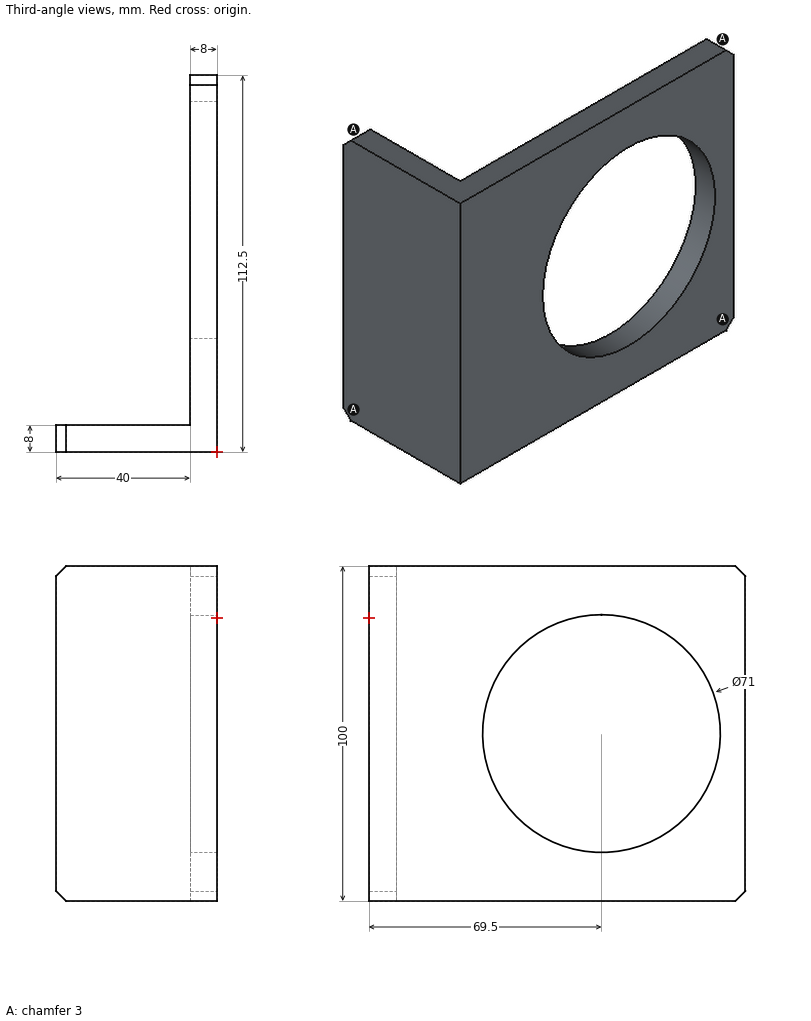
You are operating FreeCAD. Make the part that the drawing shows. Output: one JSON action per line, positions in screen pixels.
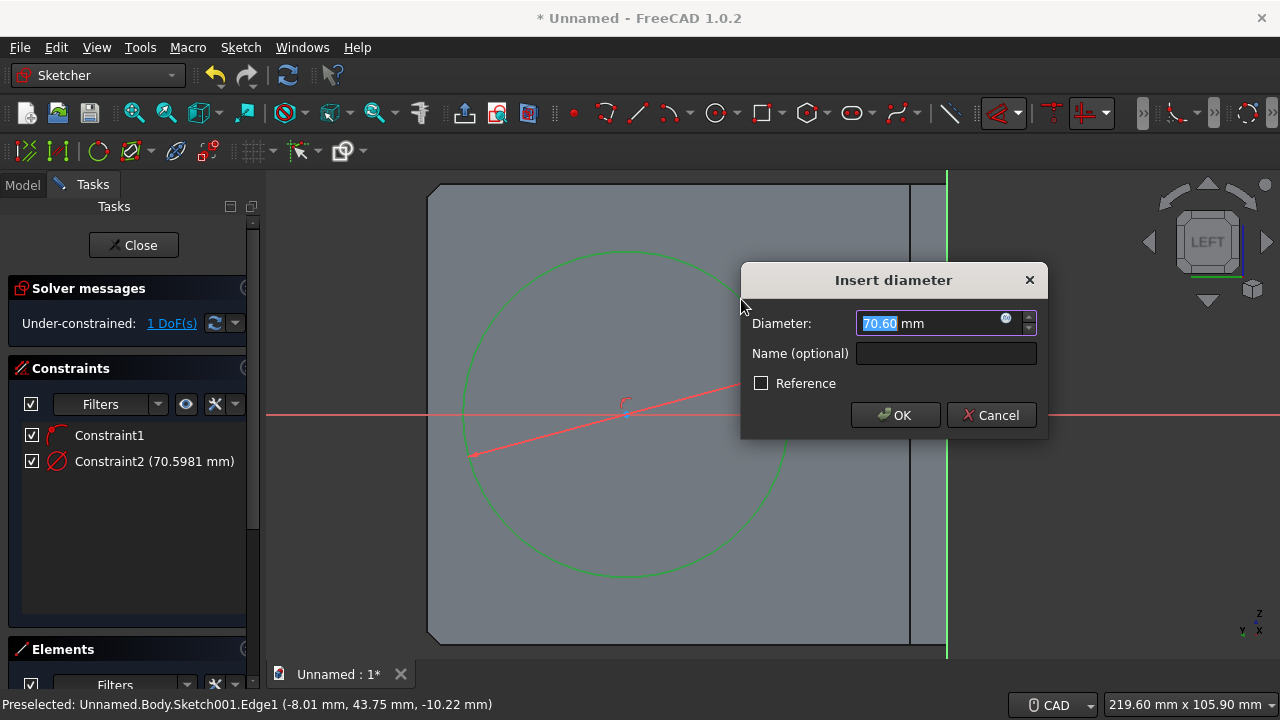
{"action": "type", "text": "71"}
{"action": "key", "text": "Return"}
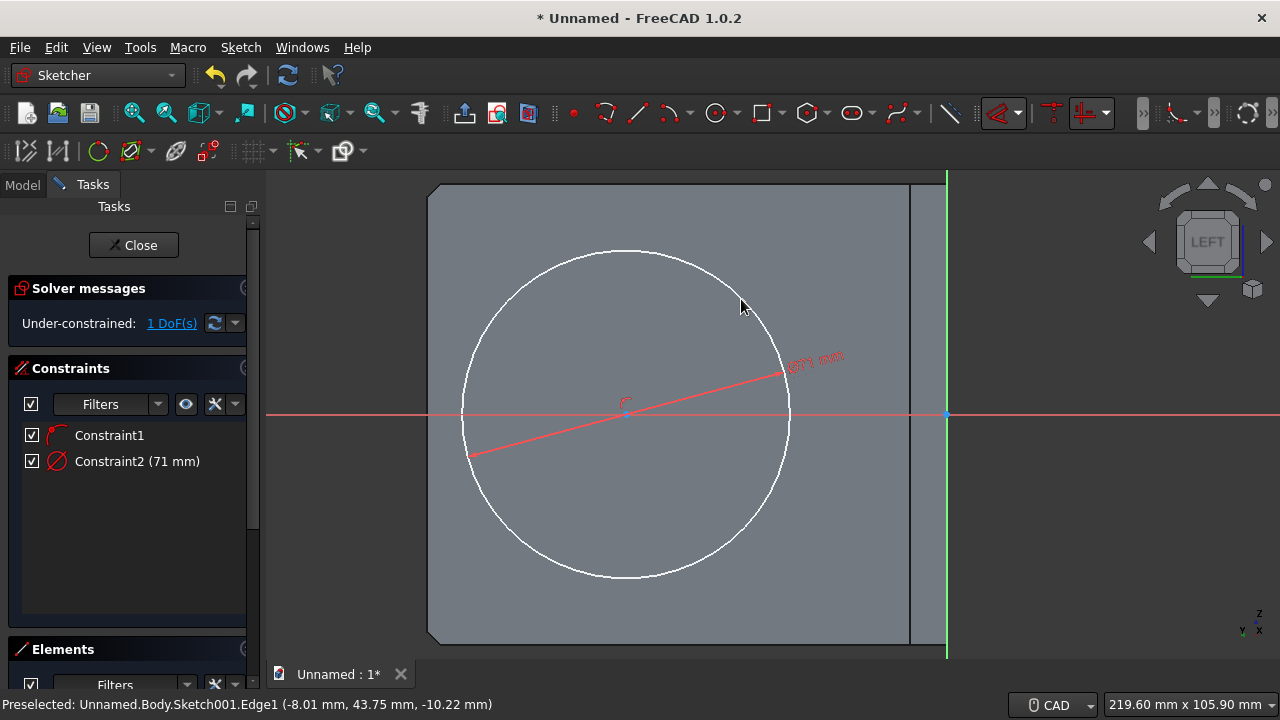
{"action": "left_click", "coordinate": [626, 414]}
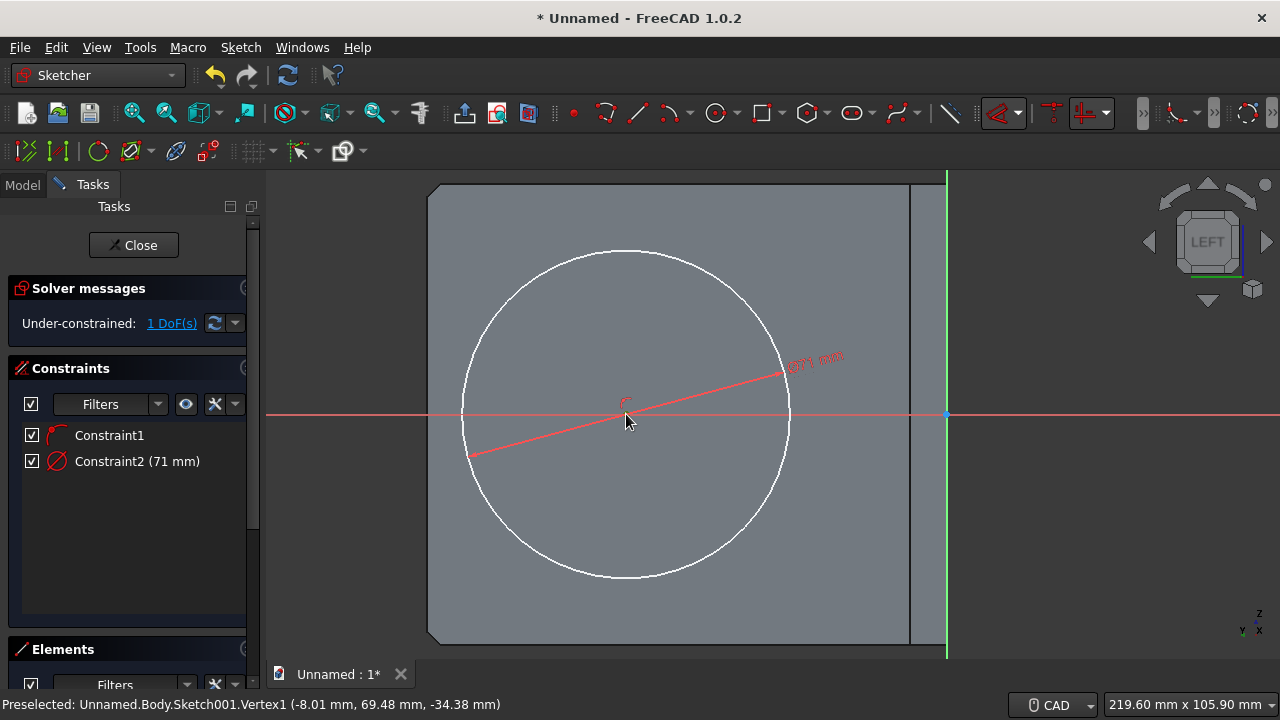
{"action": "left_click", "coordinate": [1020, 114]}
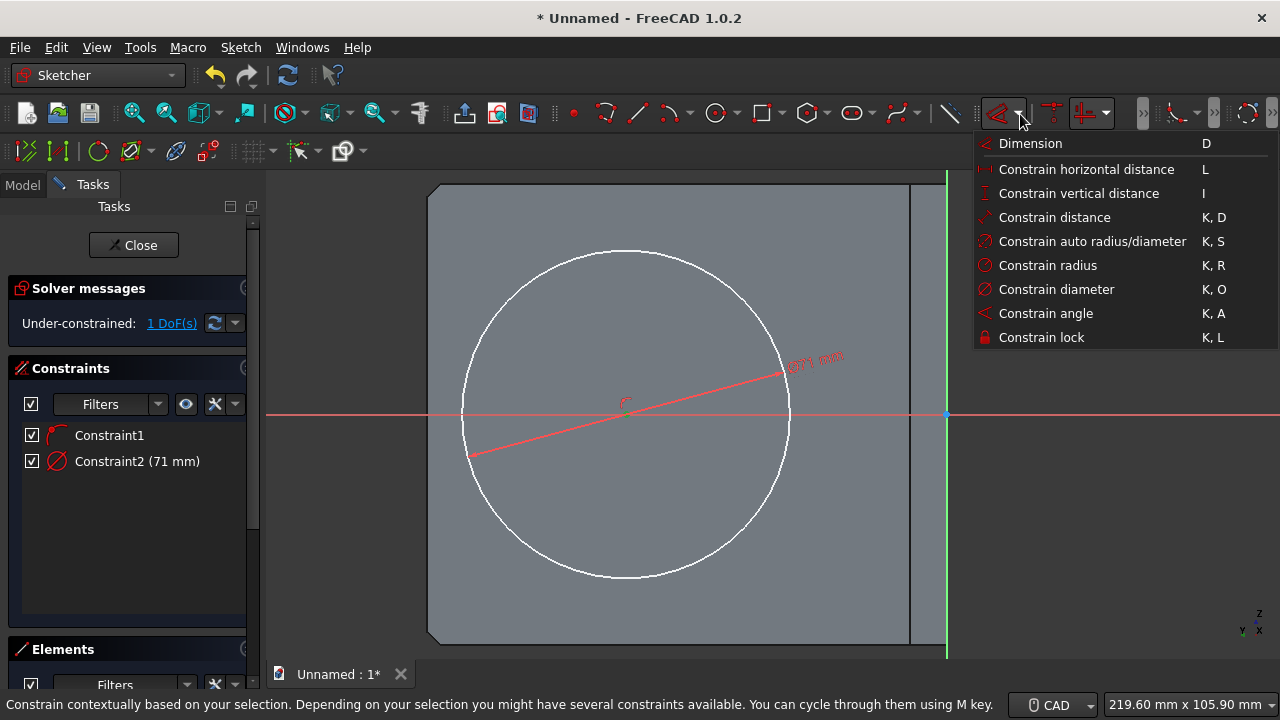
{"action": "left_click", "coordinate": [1126, 169]}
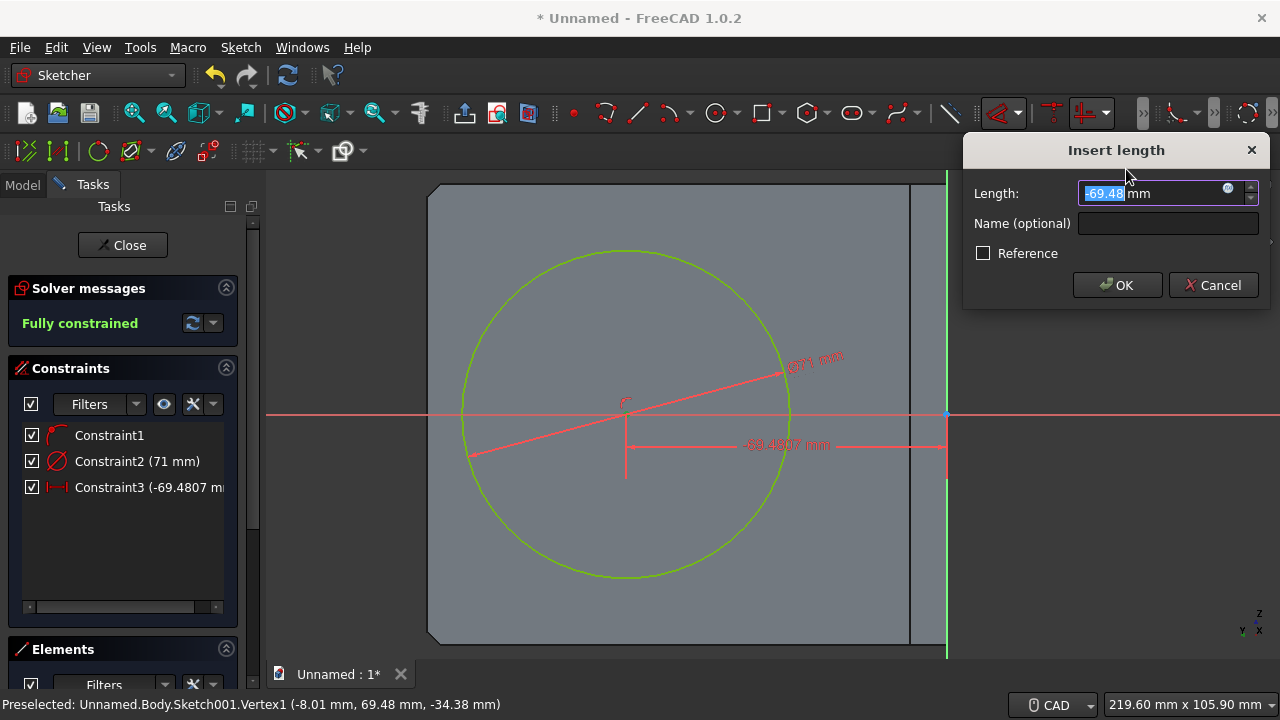
{"action": "type", "text": "-69.5"}
{"action": "key", "text": "Return"}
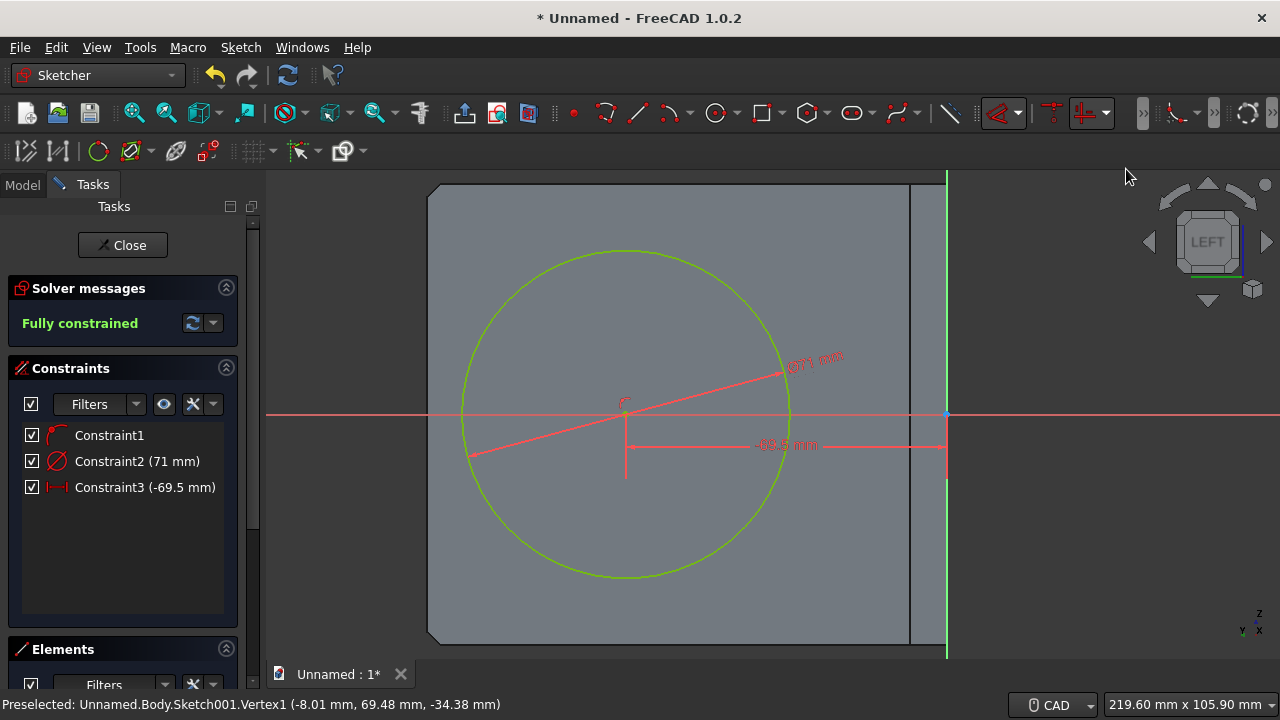
{"action": "left_click", "coordinate": [123, 245]}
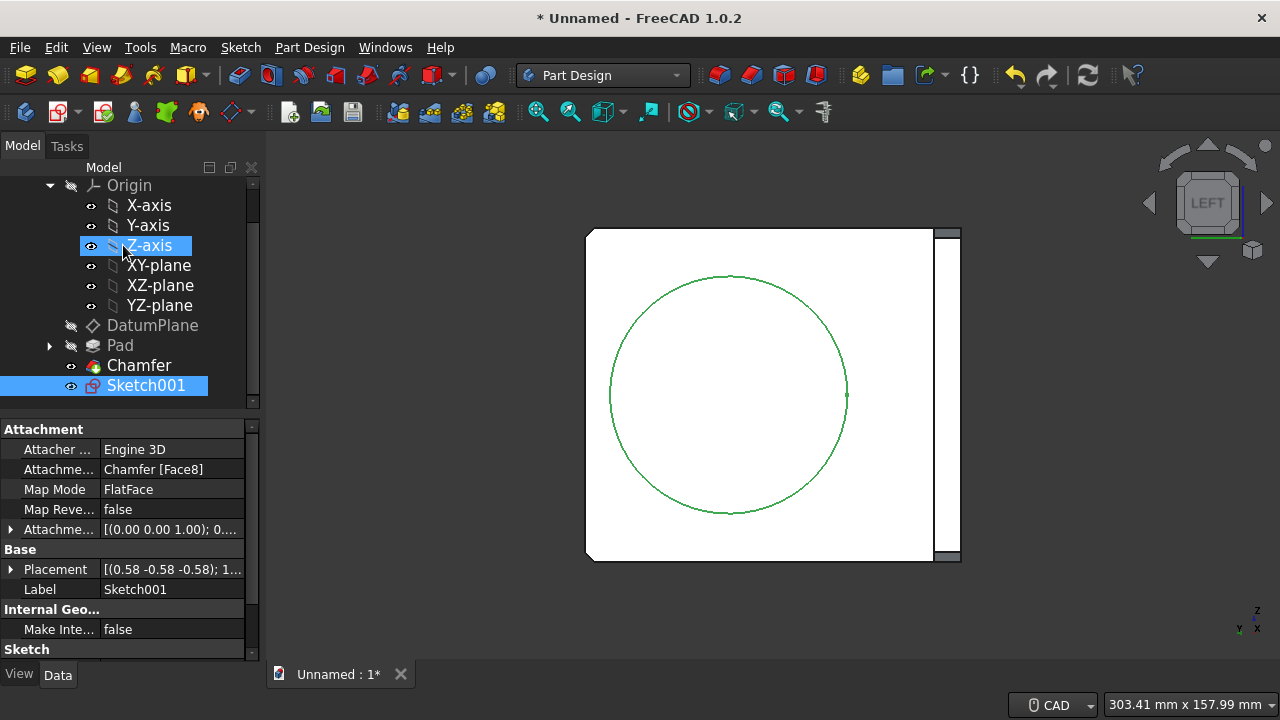
{"action": "left_click", "coordinate": [240, 76]}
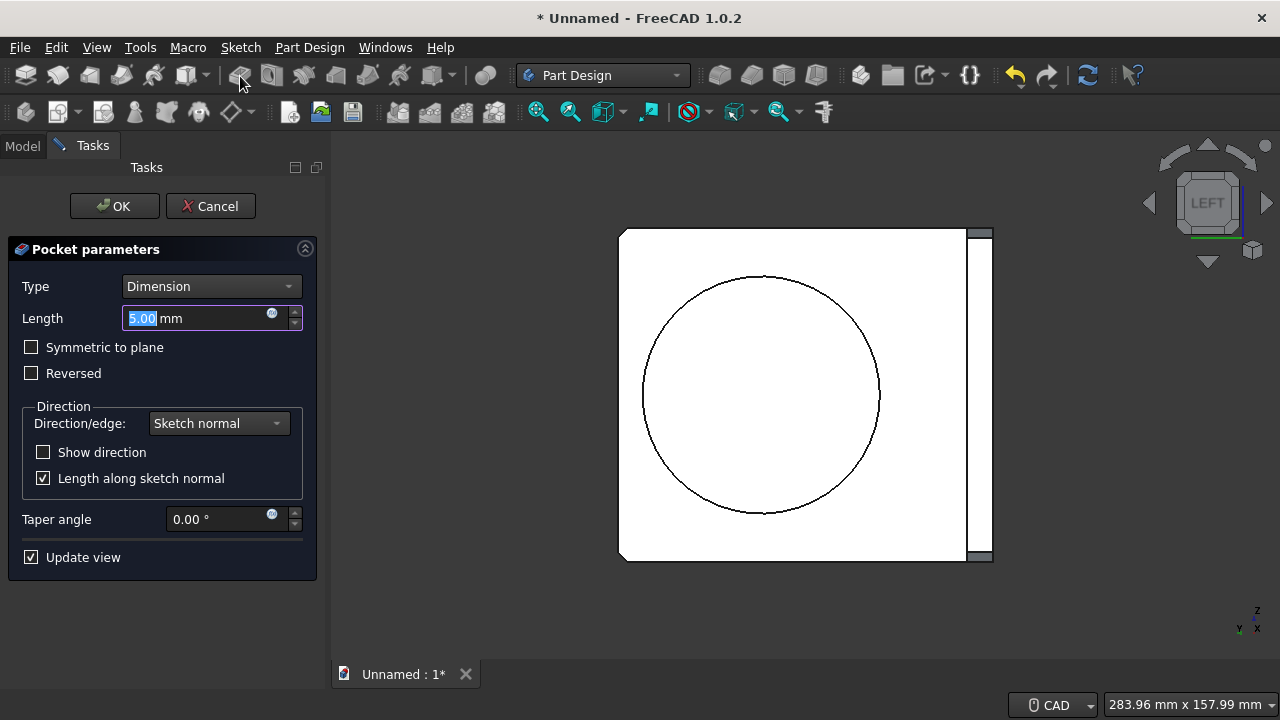
{"action": "left_click", "coordinate": [212, 286]}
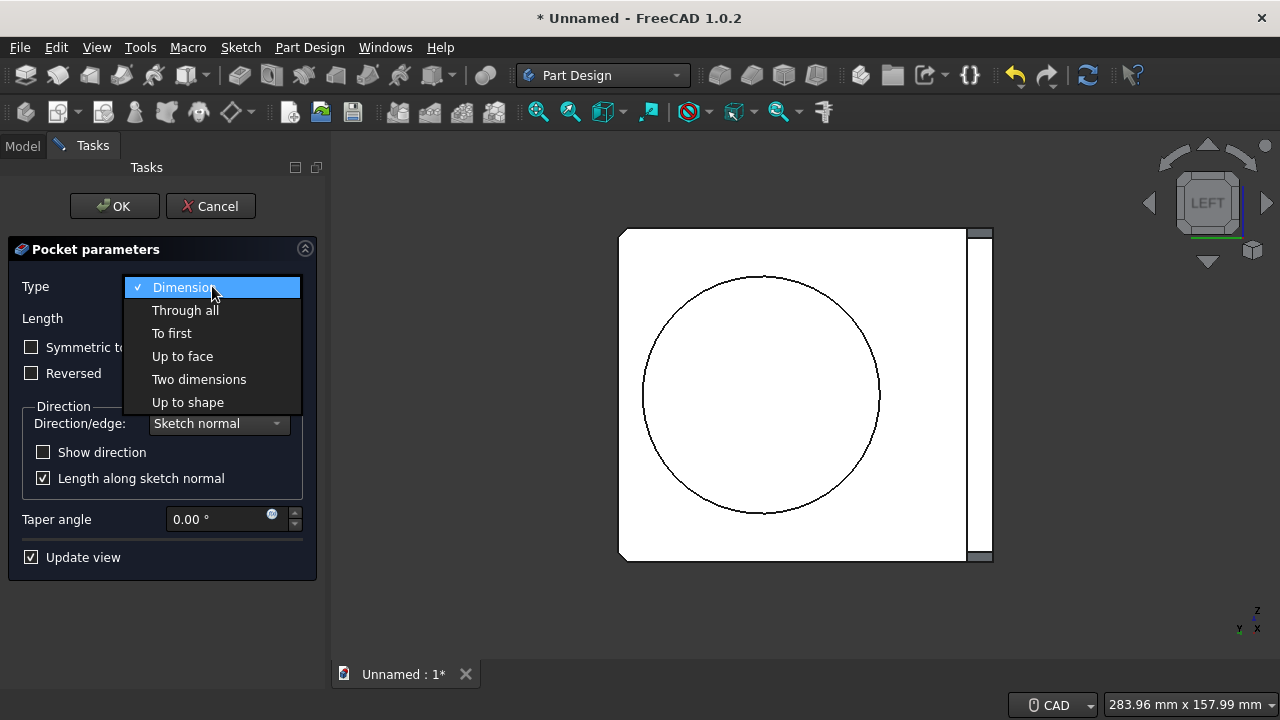
{"action": "left_click", "coordinate": [212, 334]}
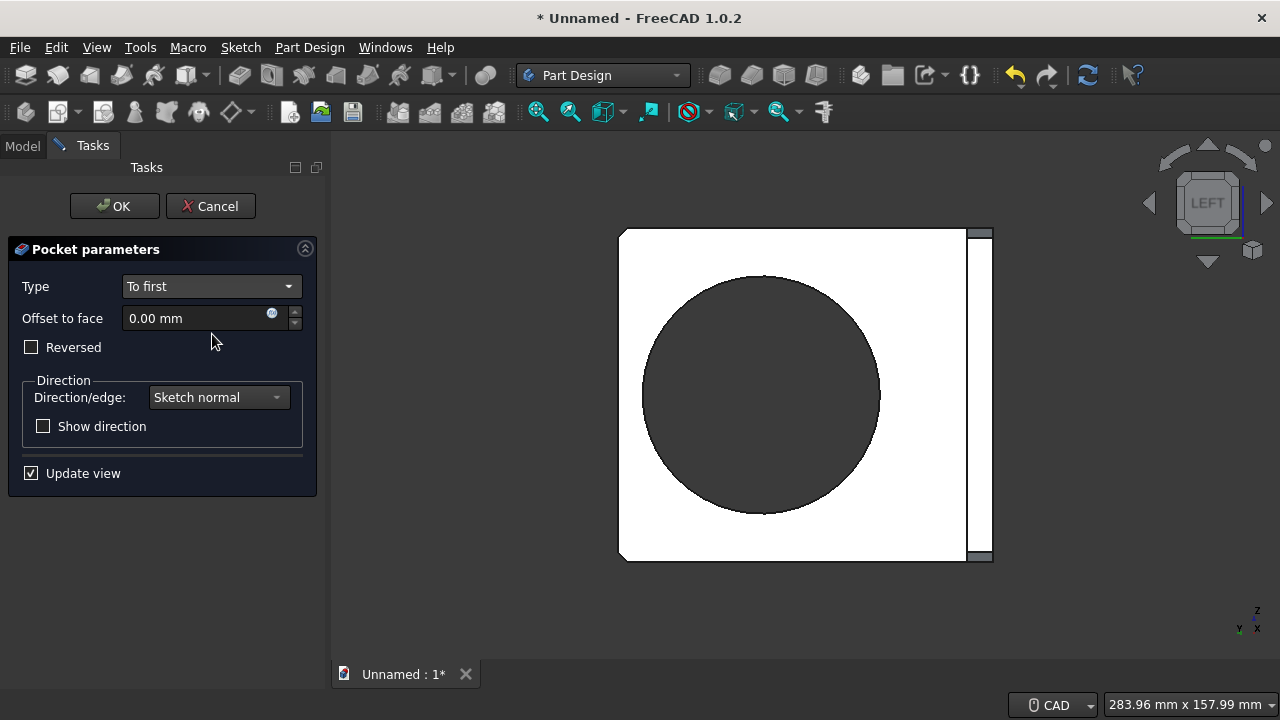
{"action": "left_click", "coordinate": [115, 206]}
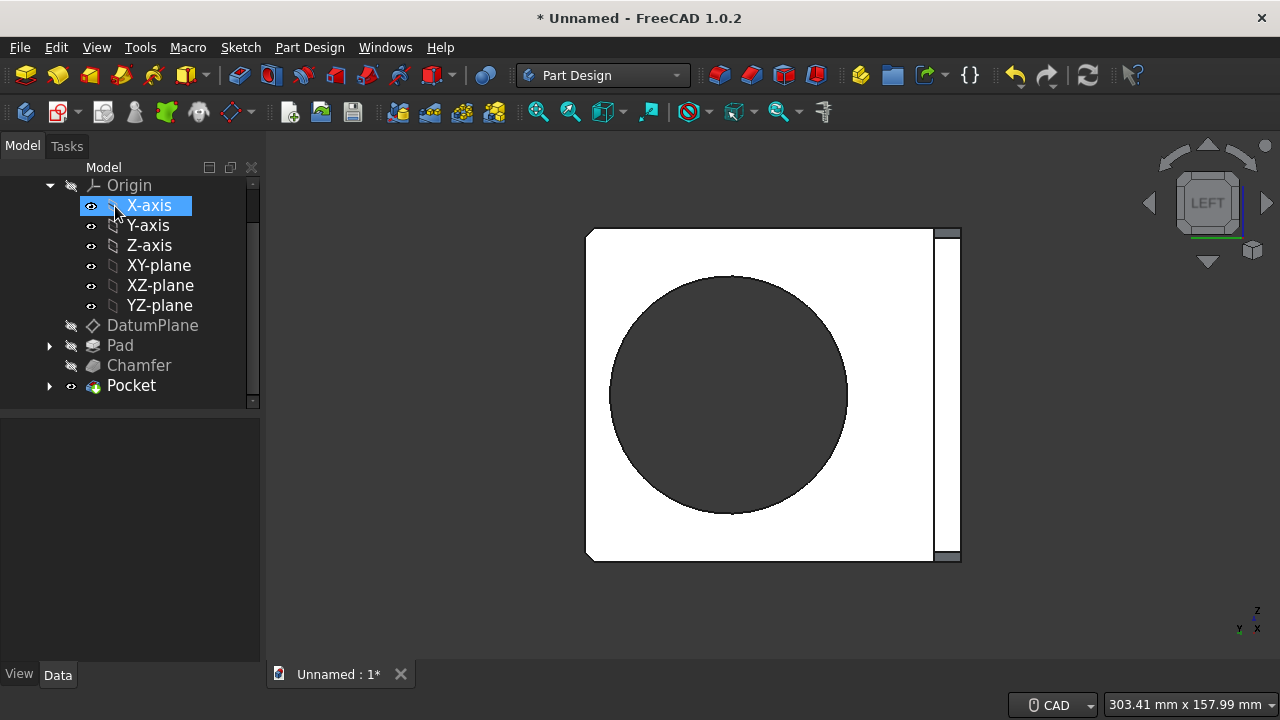
{"action": "key", "text": "0"}